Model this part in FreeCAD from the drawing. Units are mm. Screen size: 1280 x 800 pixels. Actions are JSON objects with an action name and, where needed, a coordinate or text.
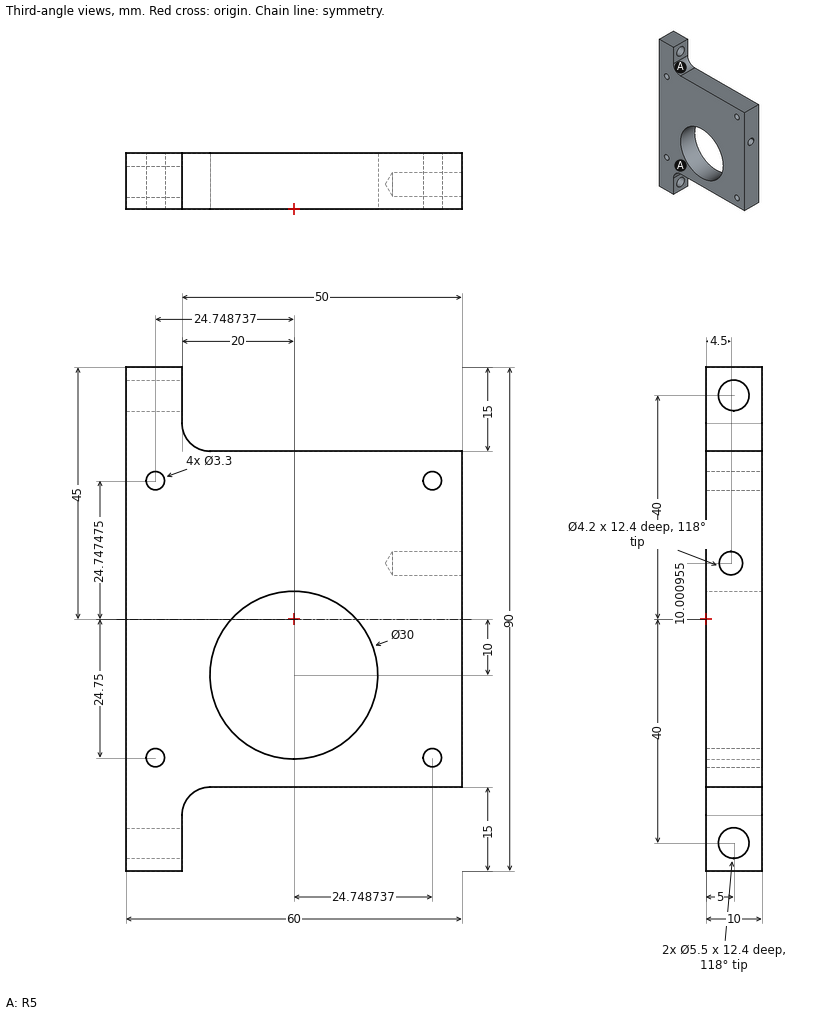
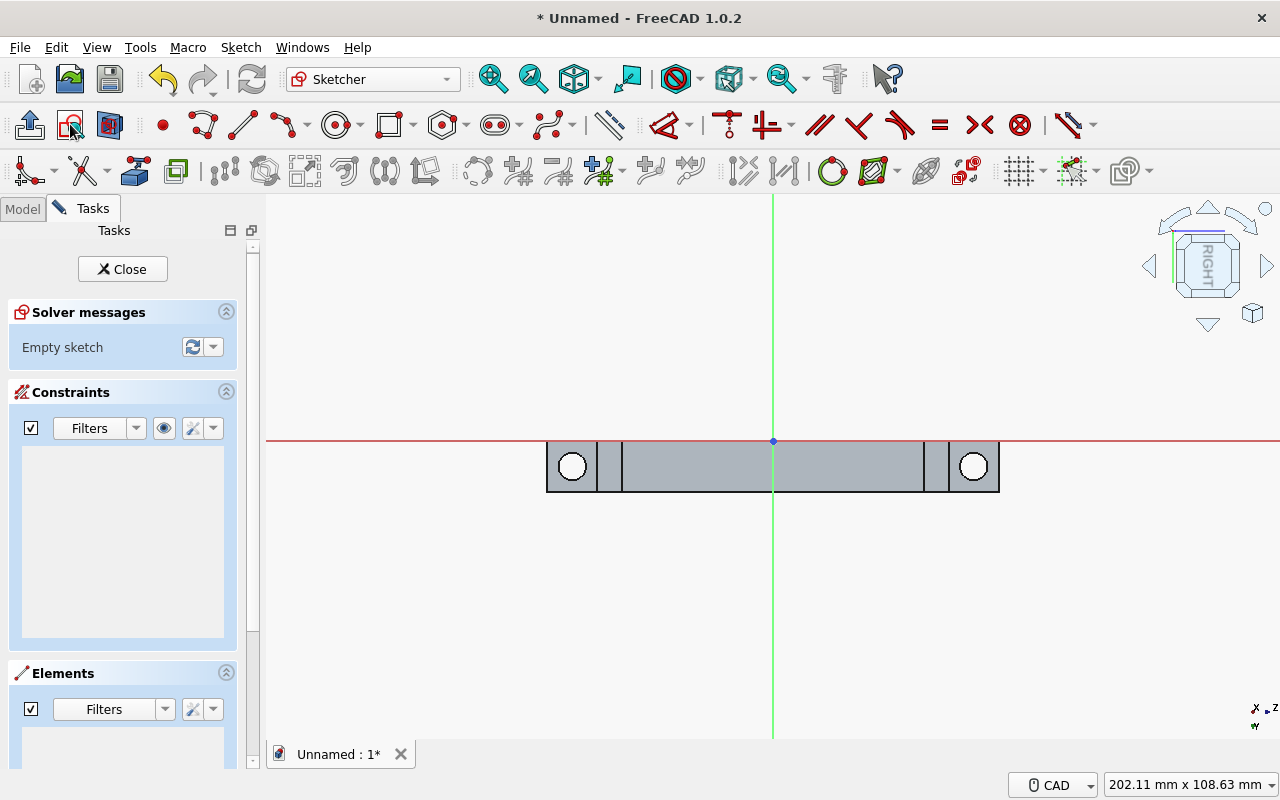
{"action": "scroll", "coordinate": [831, 464], "scroll_direction": "up", "scroll_amount": 14}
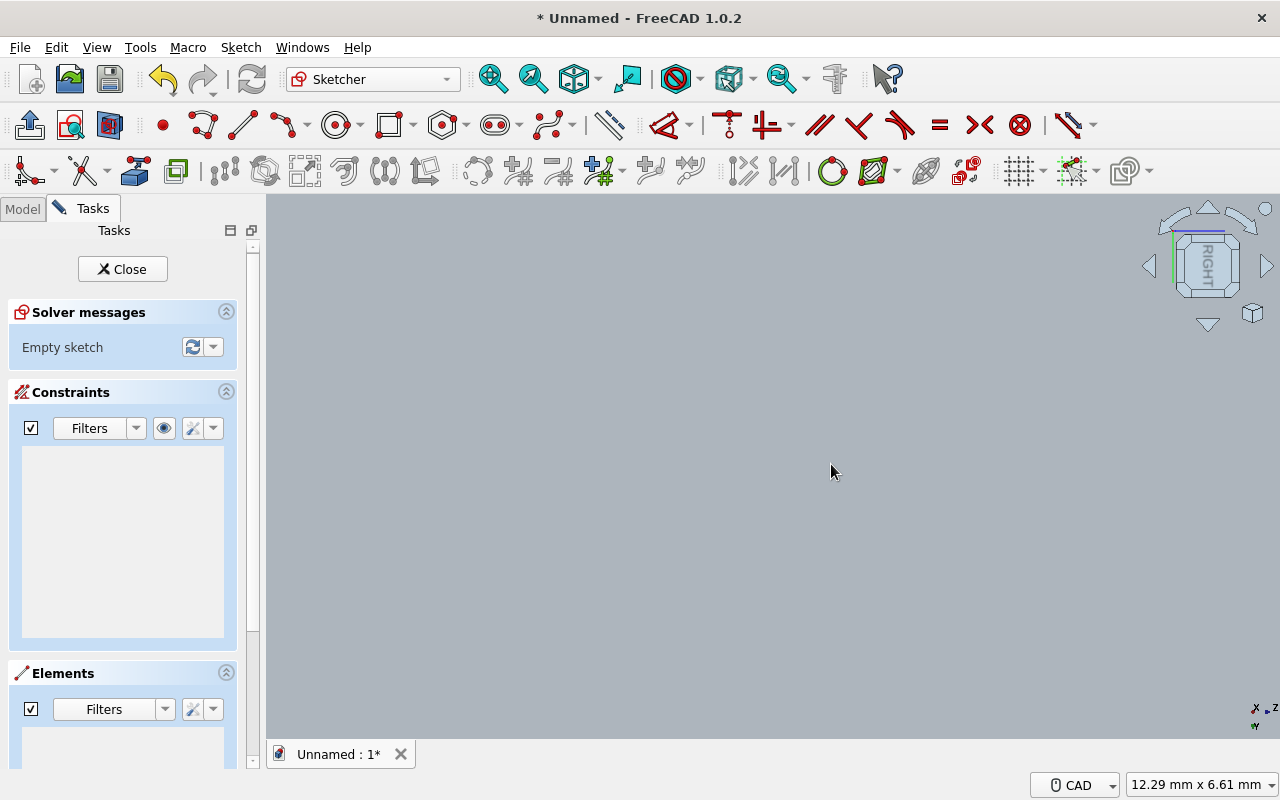
{"action": "left_click", "coordinate": [336, 126]}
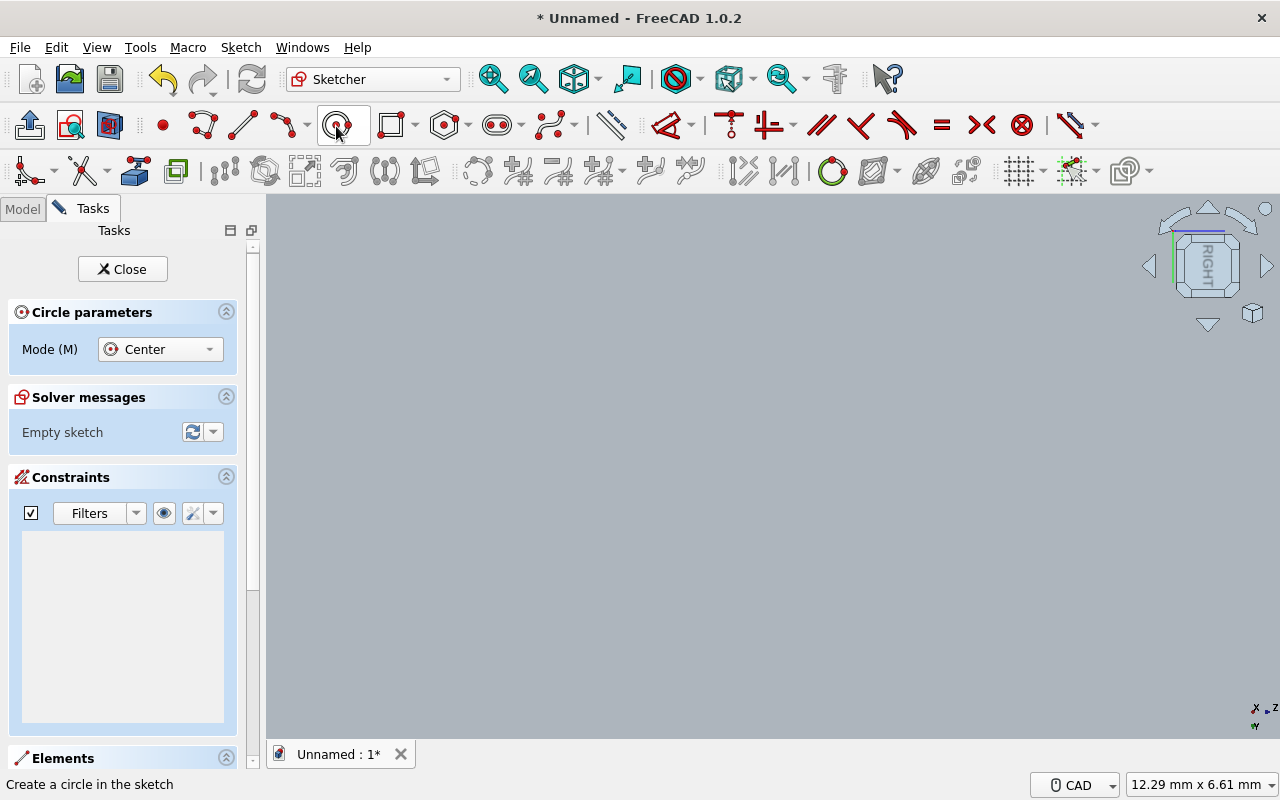
{"action": "left_click", "coordinate": [694, 456]}
{"action": "mouse_move", "coordinate": [816, 334]}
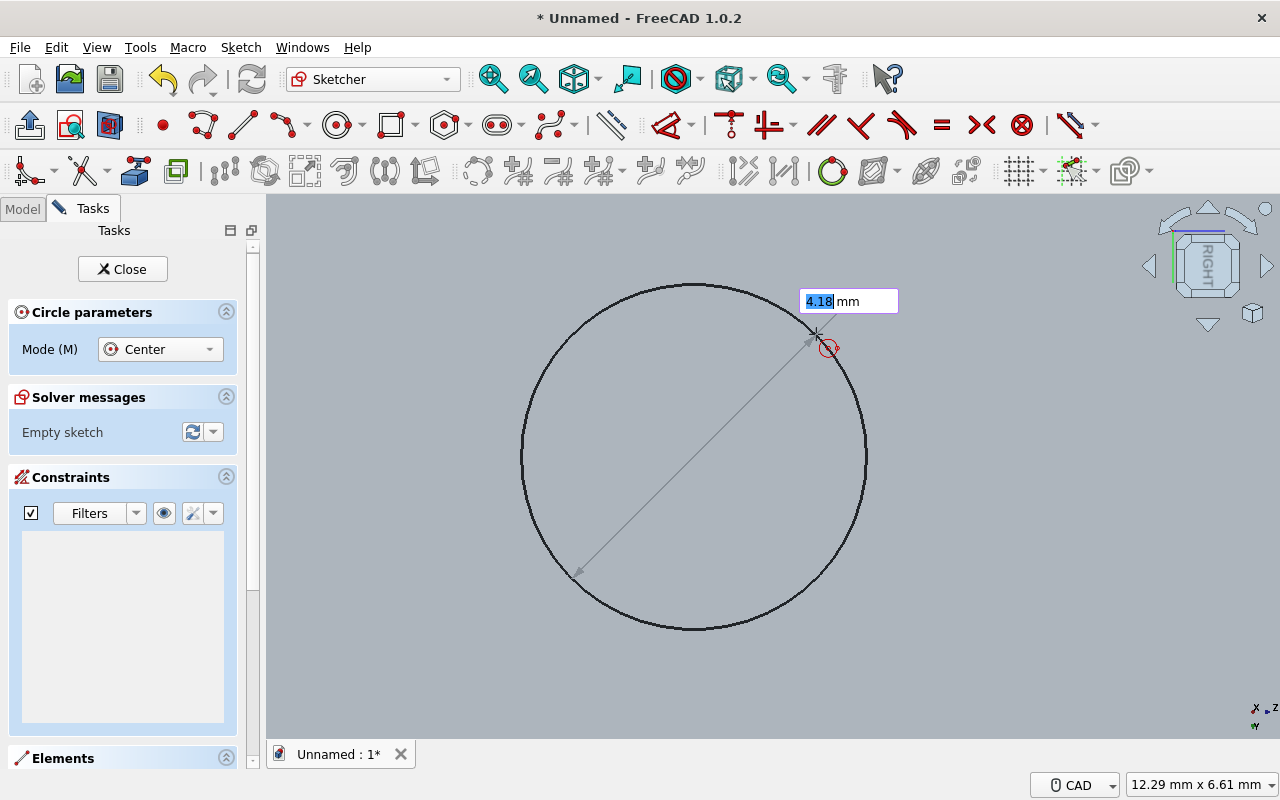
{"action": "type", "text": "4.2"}
{"action": "key", "text": "Return"}
{"action": "key", "text": "Escape"}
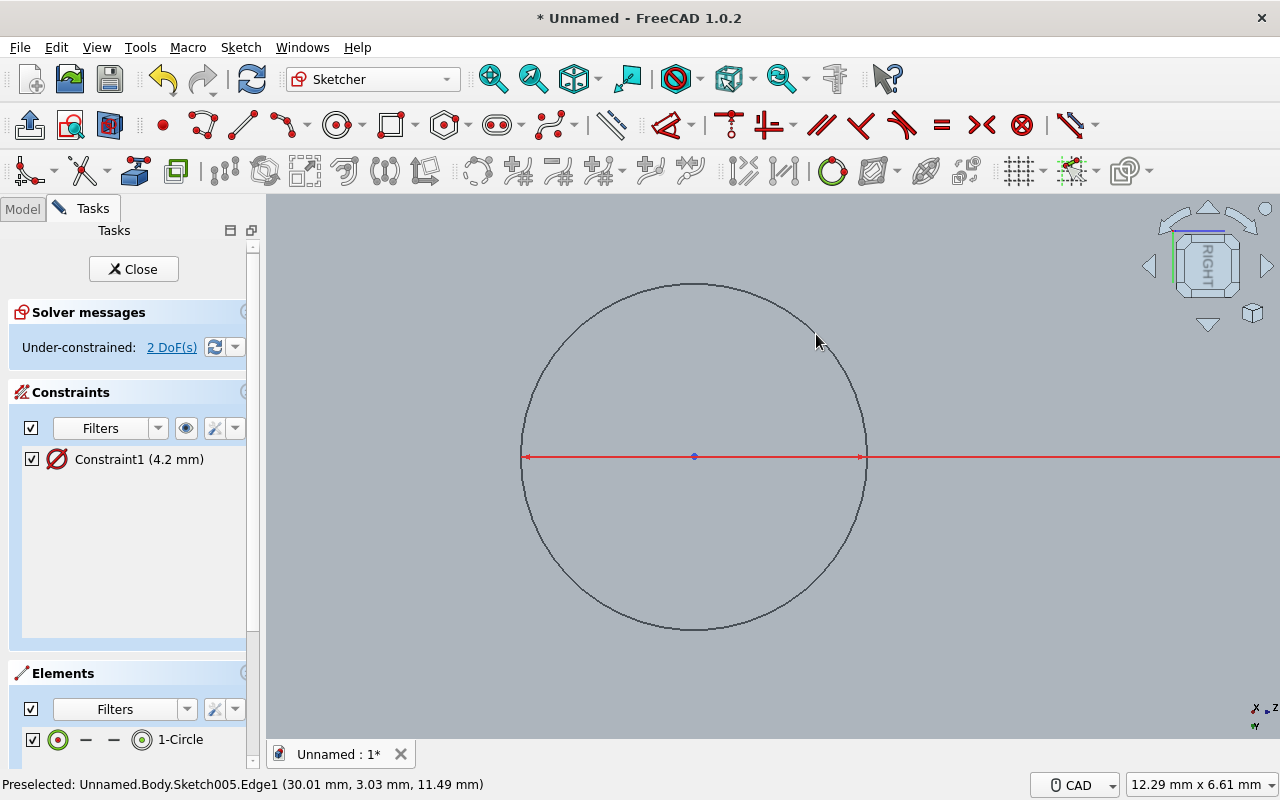
{"action": "left_click", "coordinate": [666, 126]}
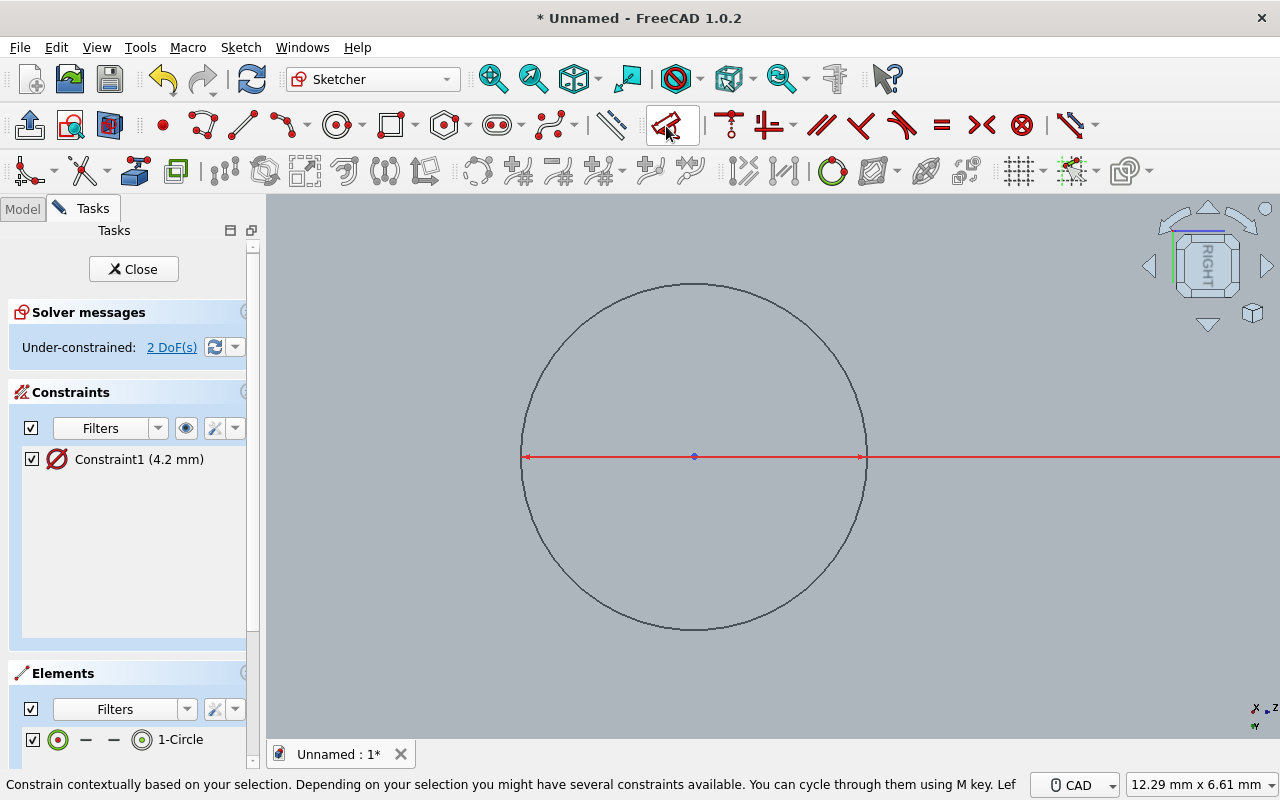
{"action": "left_click", "coordinate": [694, 457]}
{"action": "left_click", "coordinate": [728, 340]}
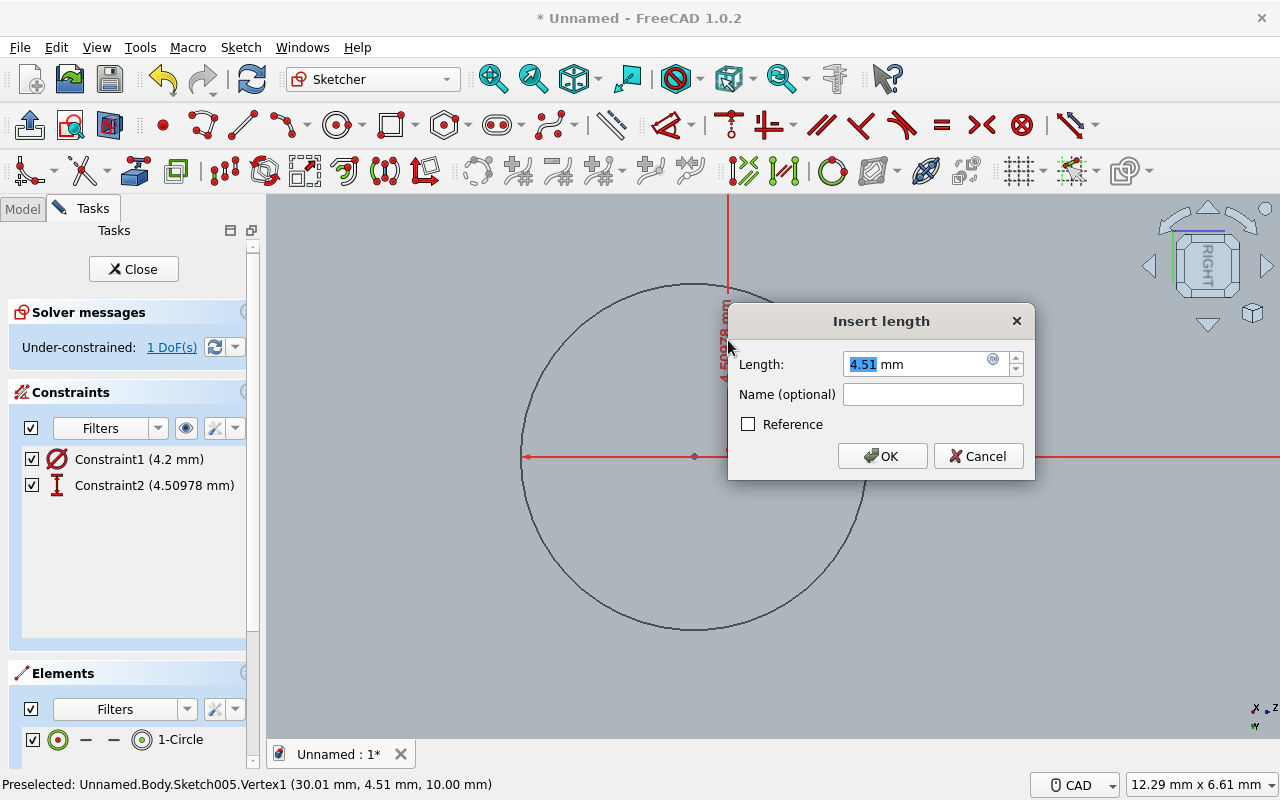
{"action": "type", "text": "4.5"}
{"action": "key", "text": "Return"}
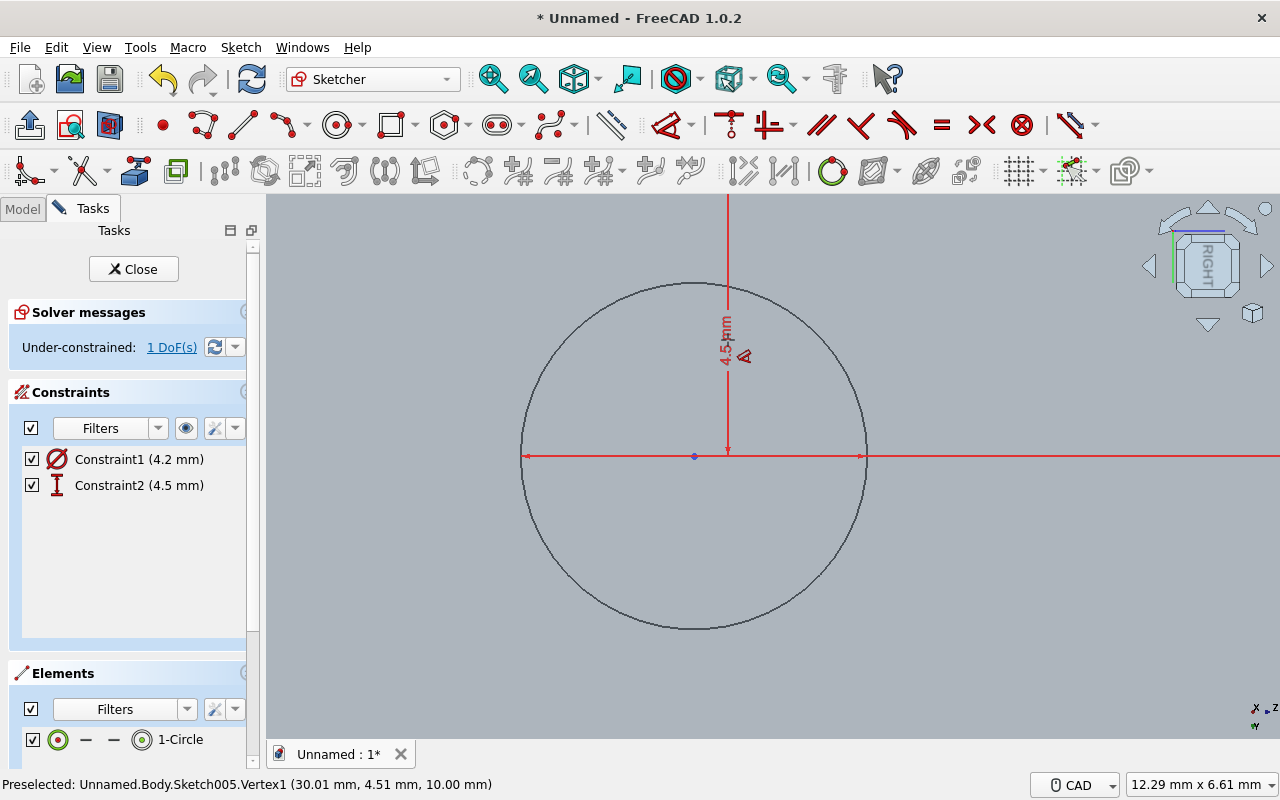
{"action": "left_click", "coordinate": [694, 456]}
{"action": "left_click", "coordinate": [494, 490]}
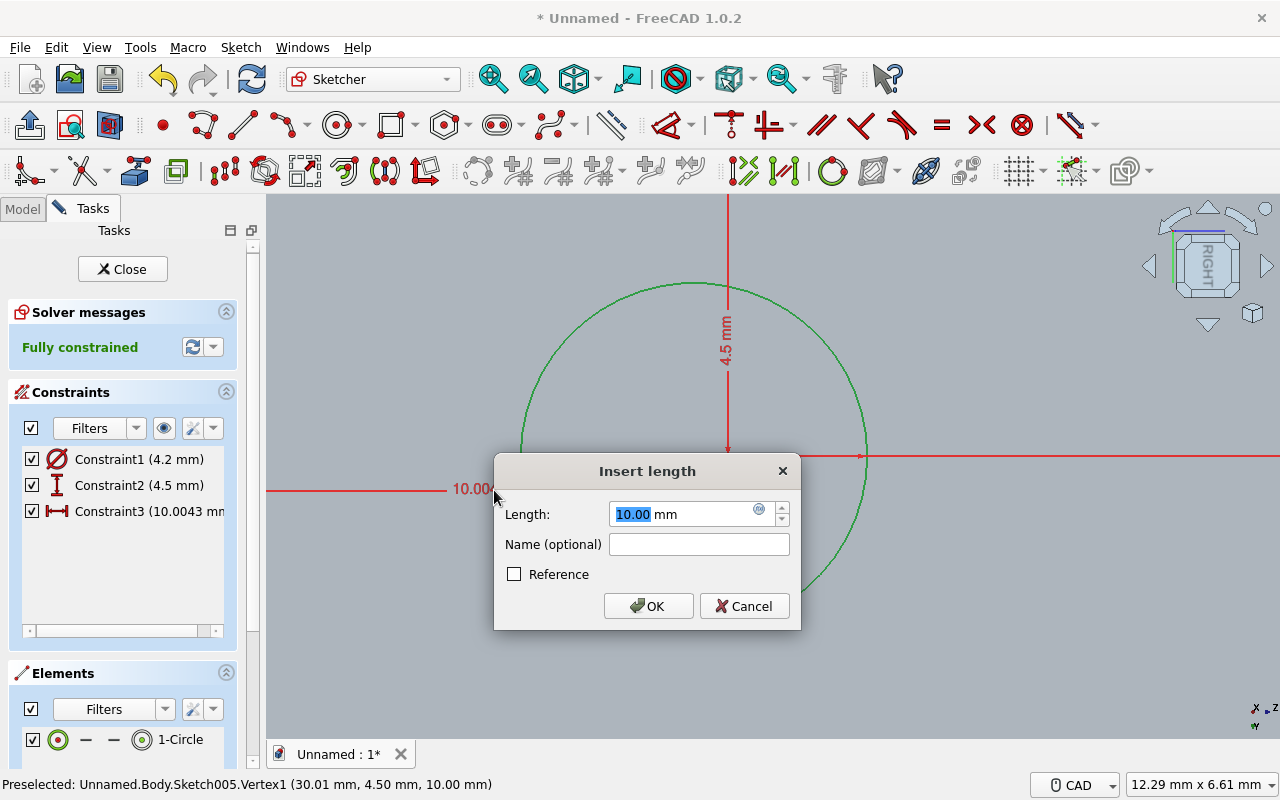
{"action": "type", "text": "10.000955"}
{"action": "key", "text": "Return"}
{"action": "key", "text": "Escape"}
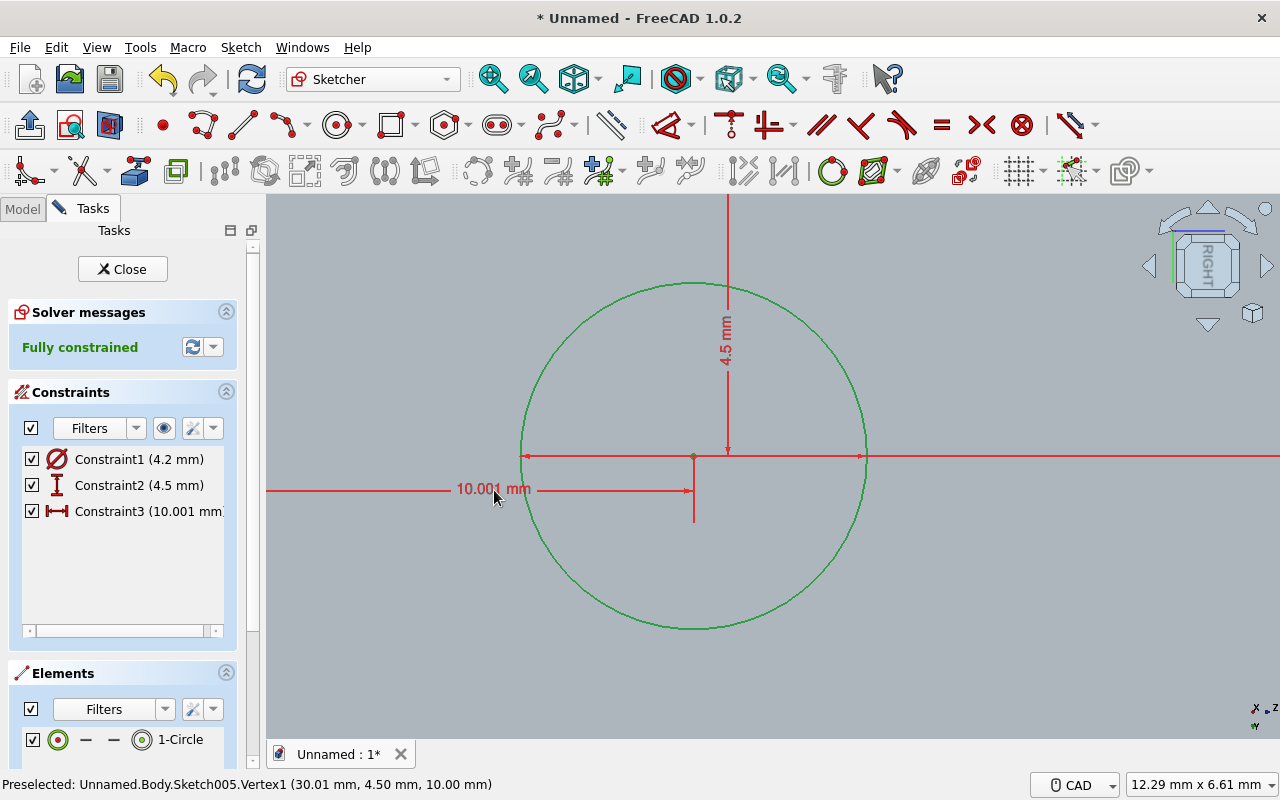
{"action": "left_click", "coordinate": [123, 269]}